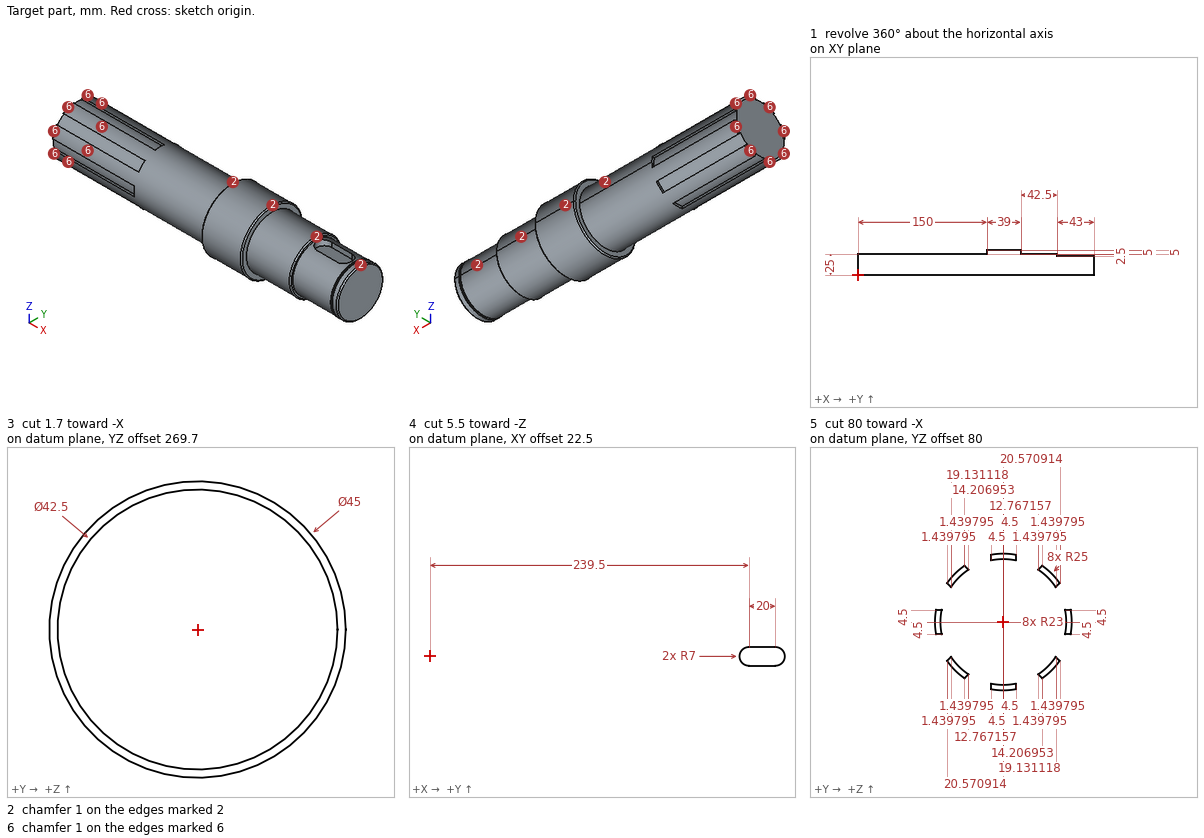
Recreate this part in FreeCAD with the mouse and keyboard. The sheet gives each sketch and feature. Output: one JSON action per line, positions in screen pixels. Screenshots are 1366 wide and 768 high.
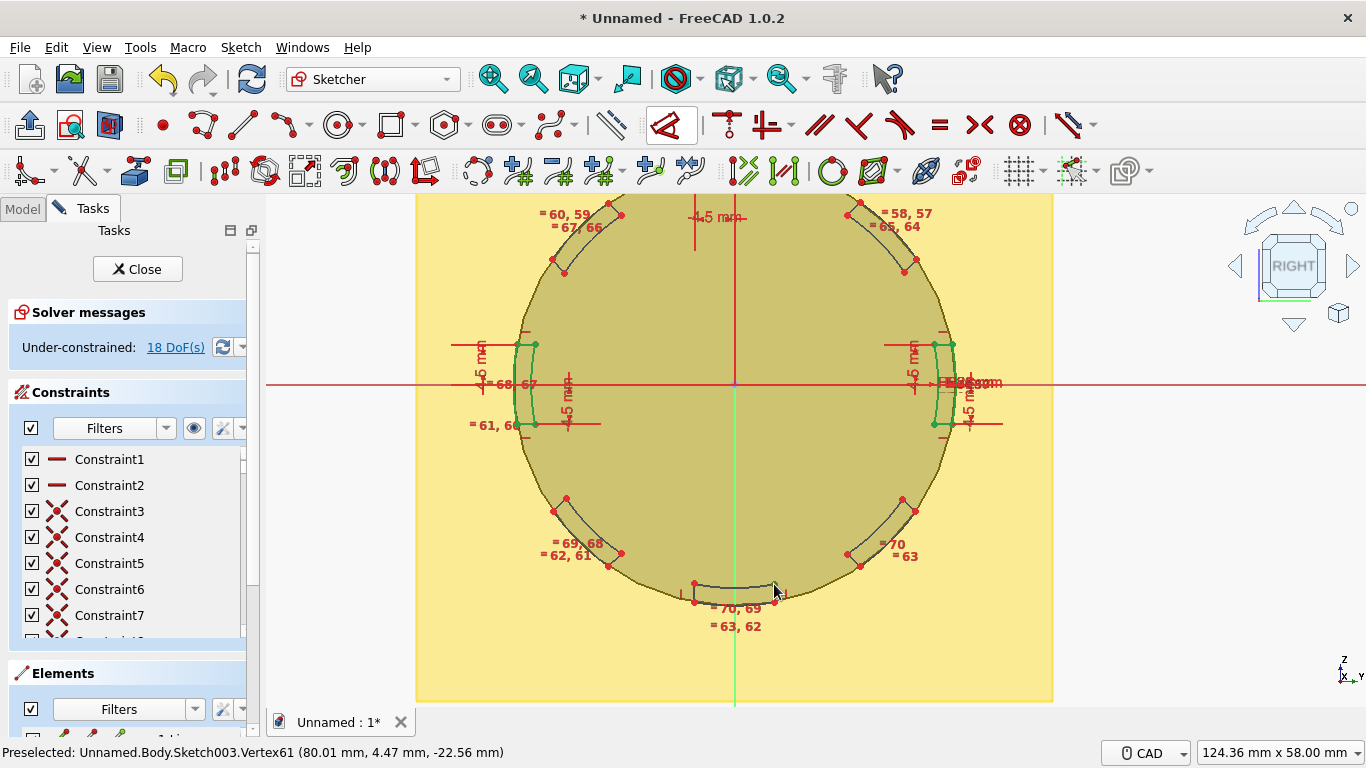
{"action": "key", "text": "l"}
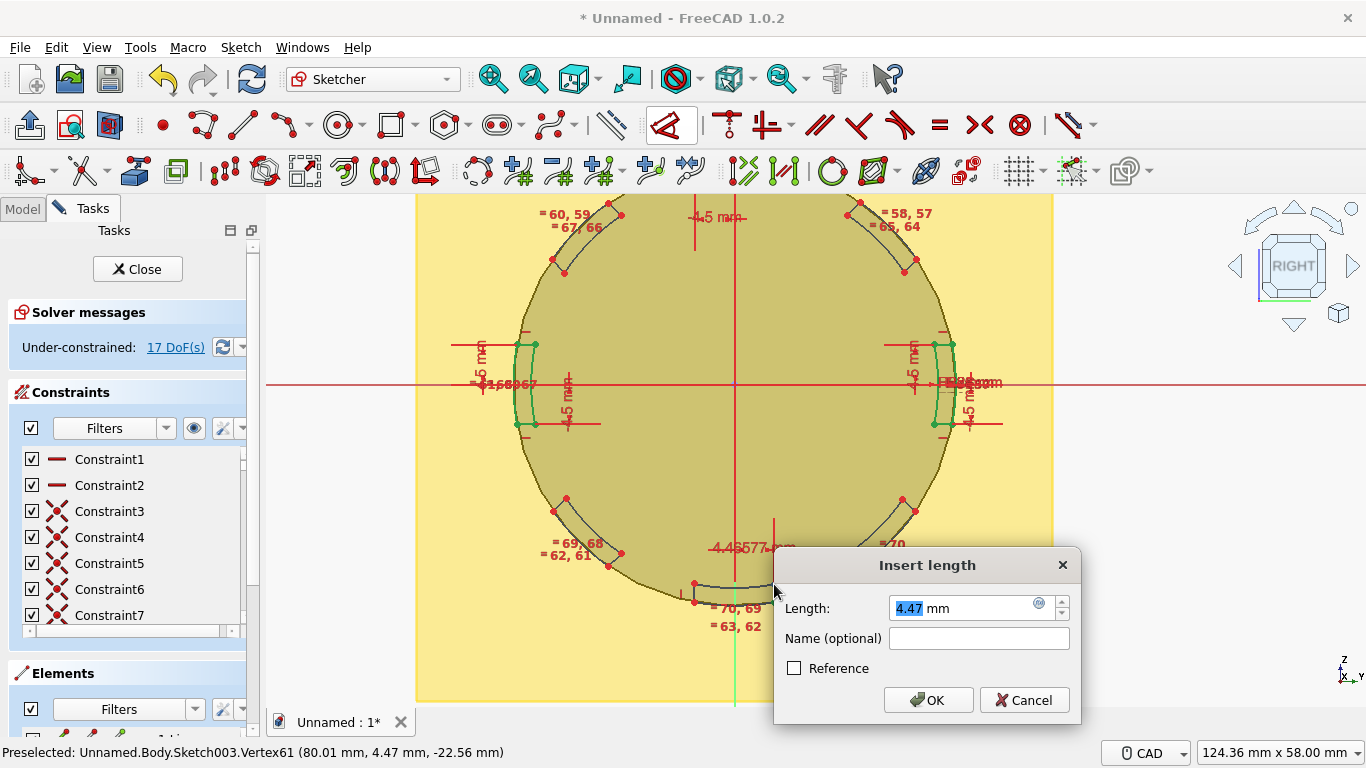
{"action": "type", "text": "4.5"}
{"action": "key", "text": "Return"}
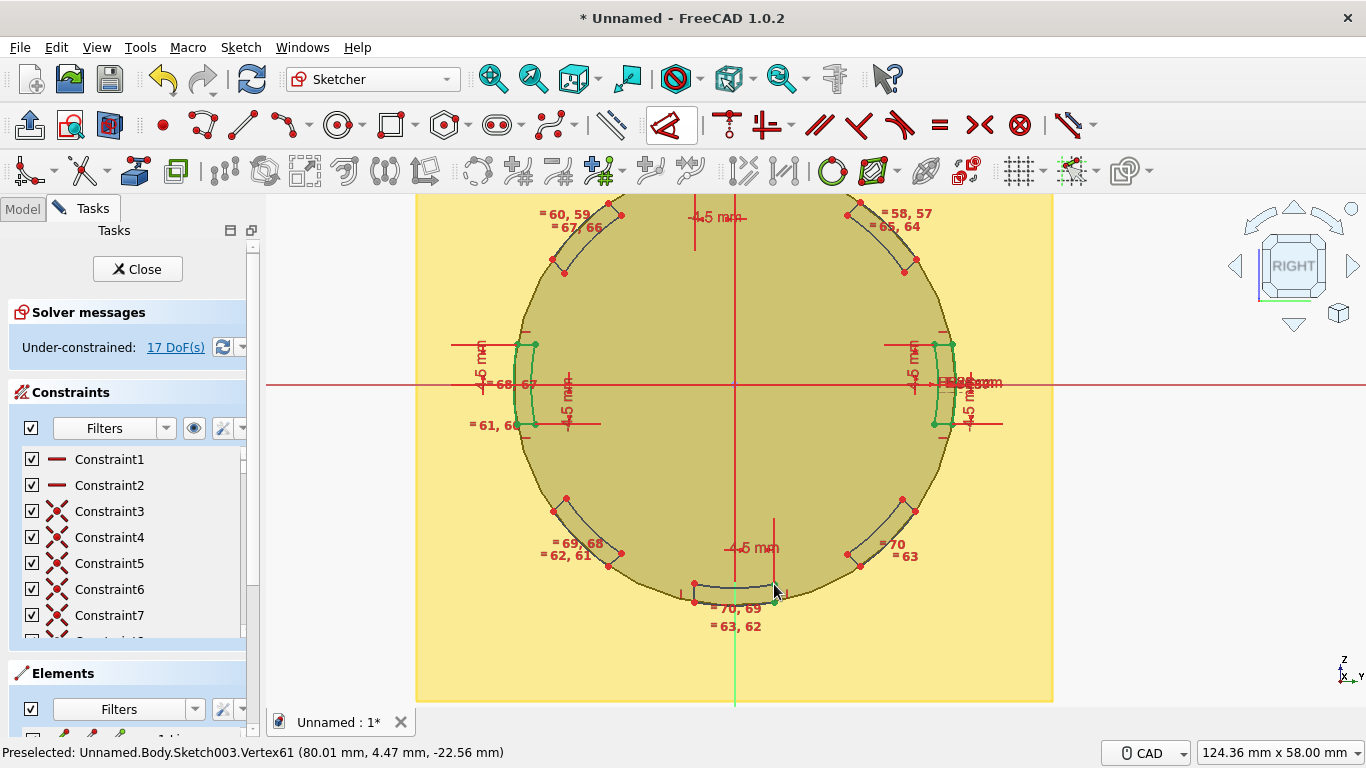
{"action": "left_click", "coordinate": [694, 602]}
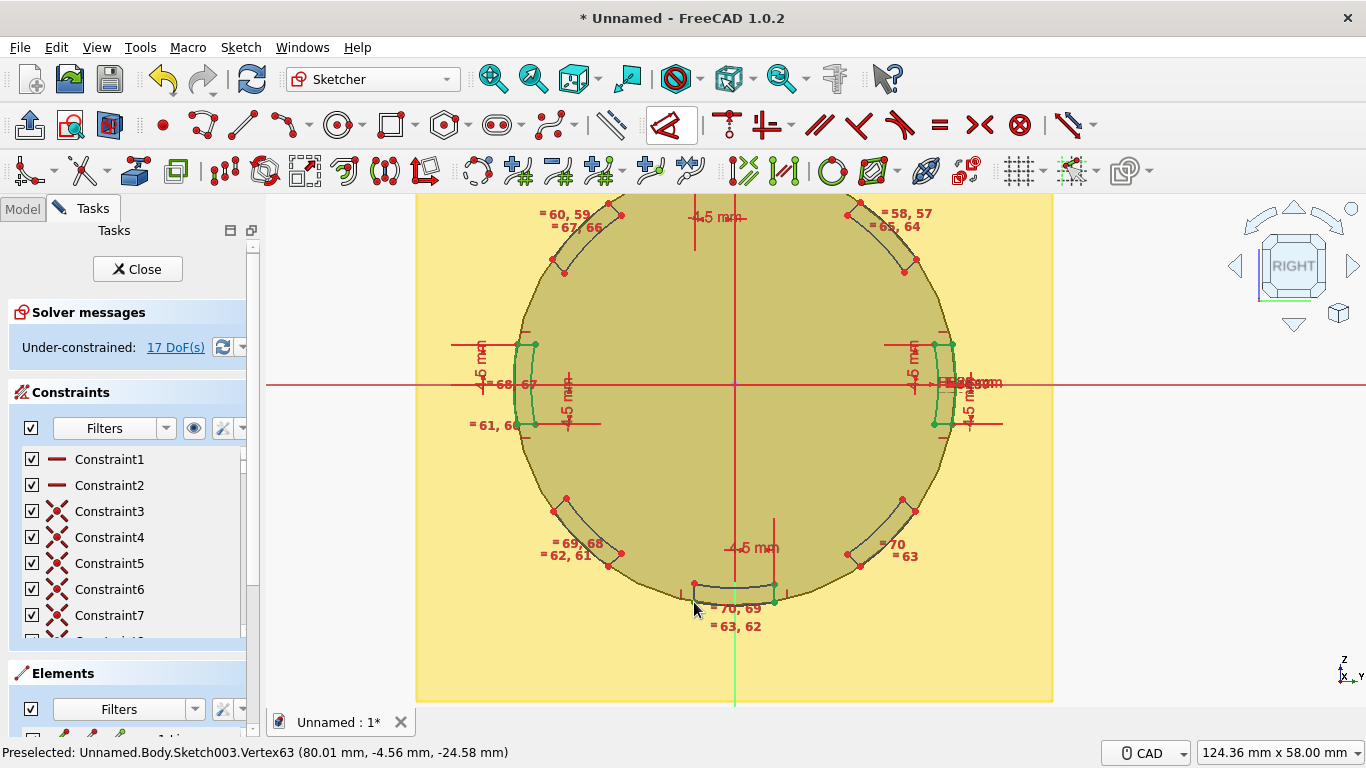
{"action": "key", "text": "l"}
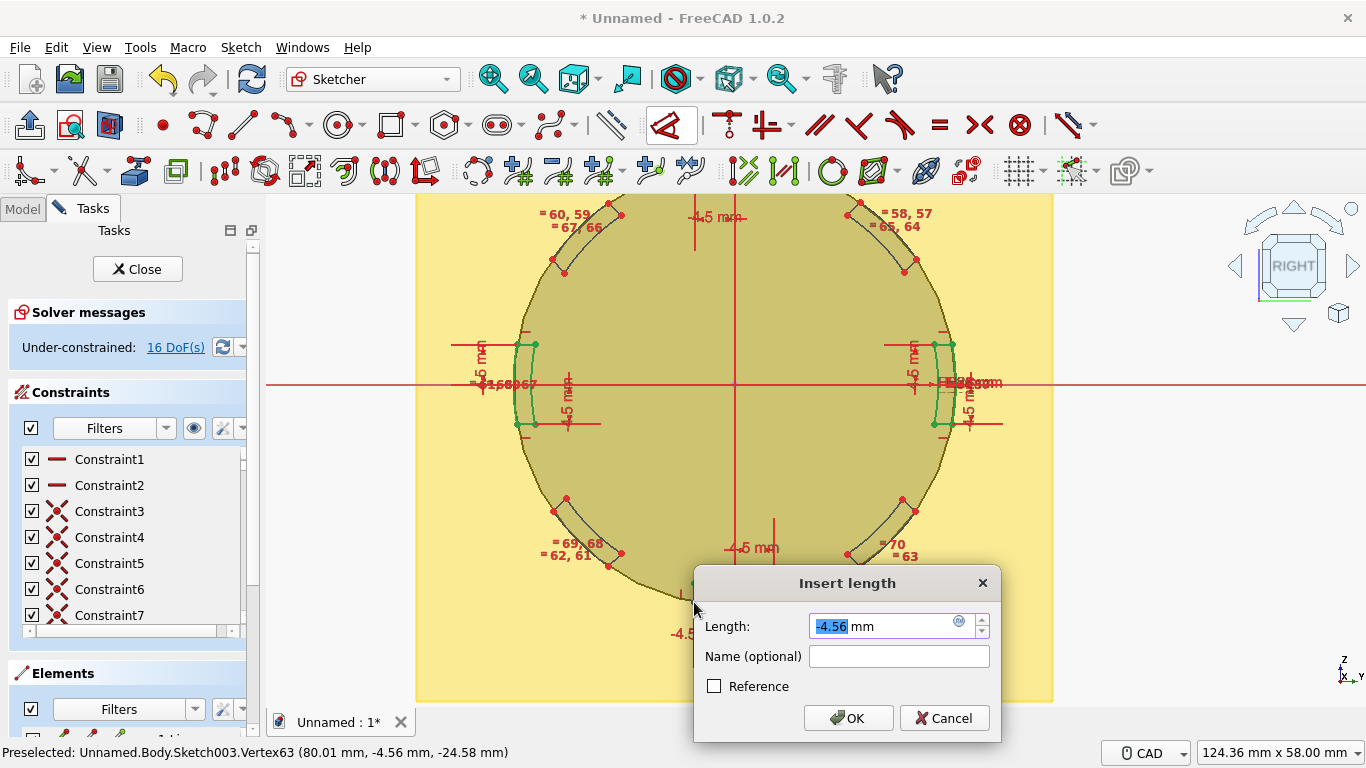
{"action": "type", "text": "-4.5"}
{"action": "key", "text": "Return"}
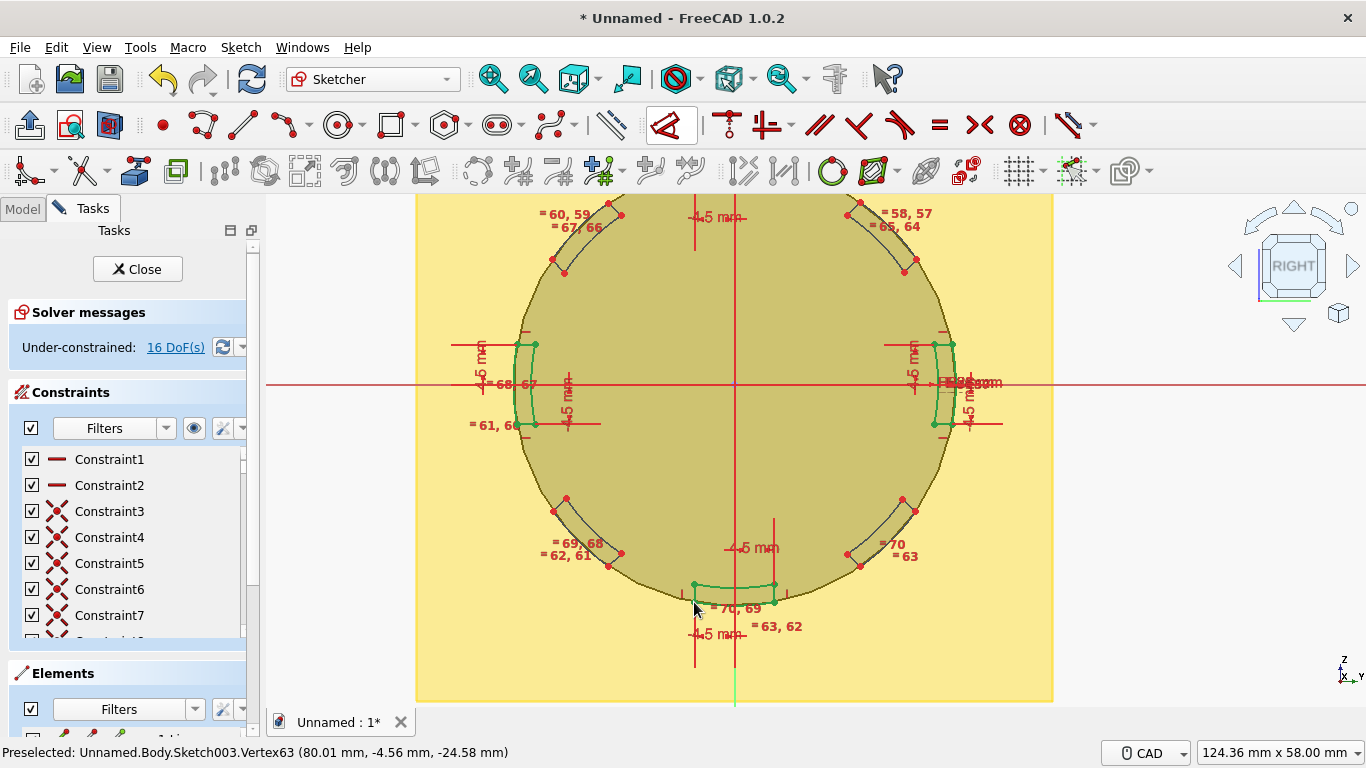
{"action": "scroll", "coordinate": [774, 585], "scroll_direction": "down", "scroll_amount": 2}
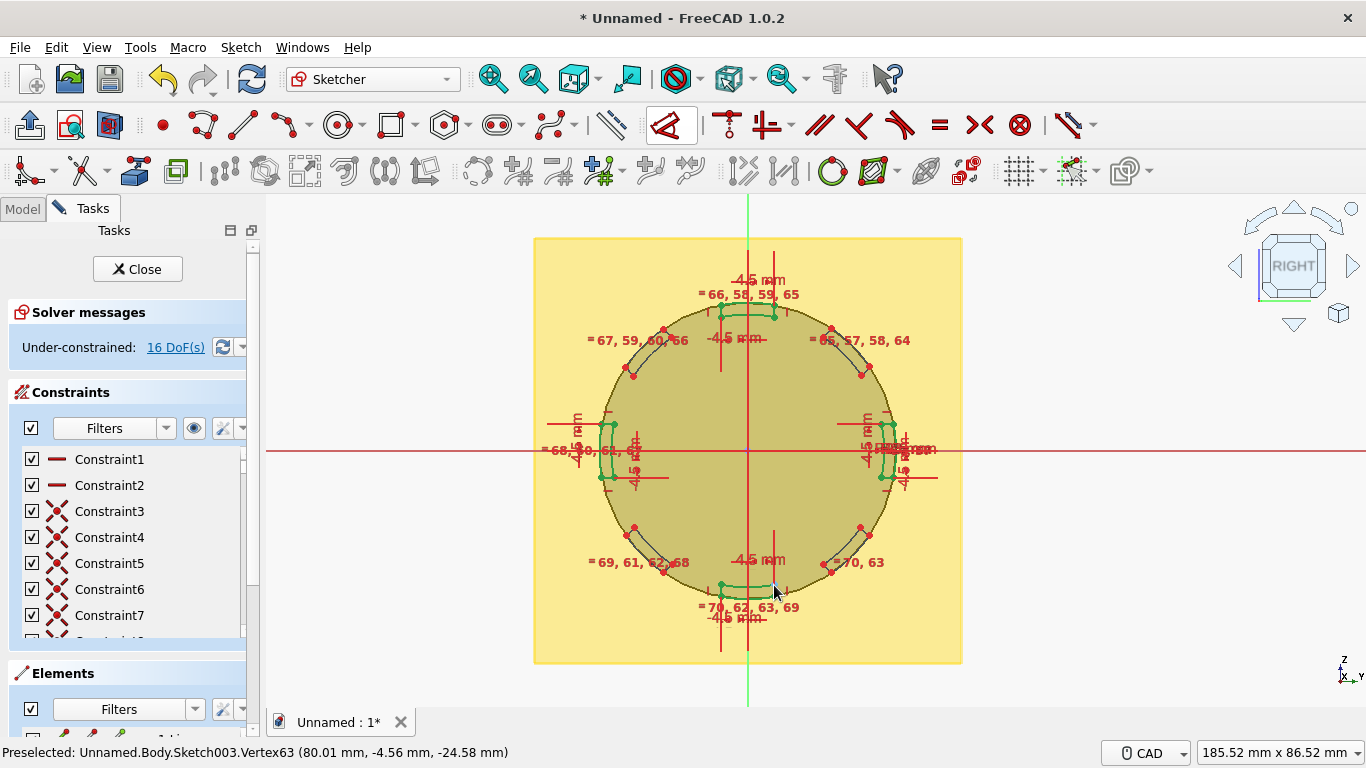
{"action": "scroll", "coordinate": [828, 333], "scroll_direction": "up", "scroll_amount": 8}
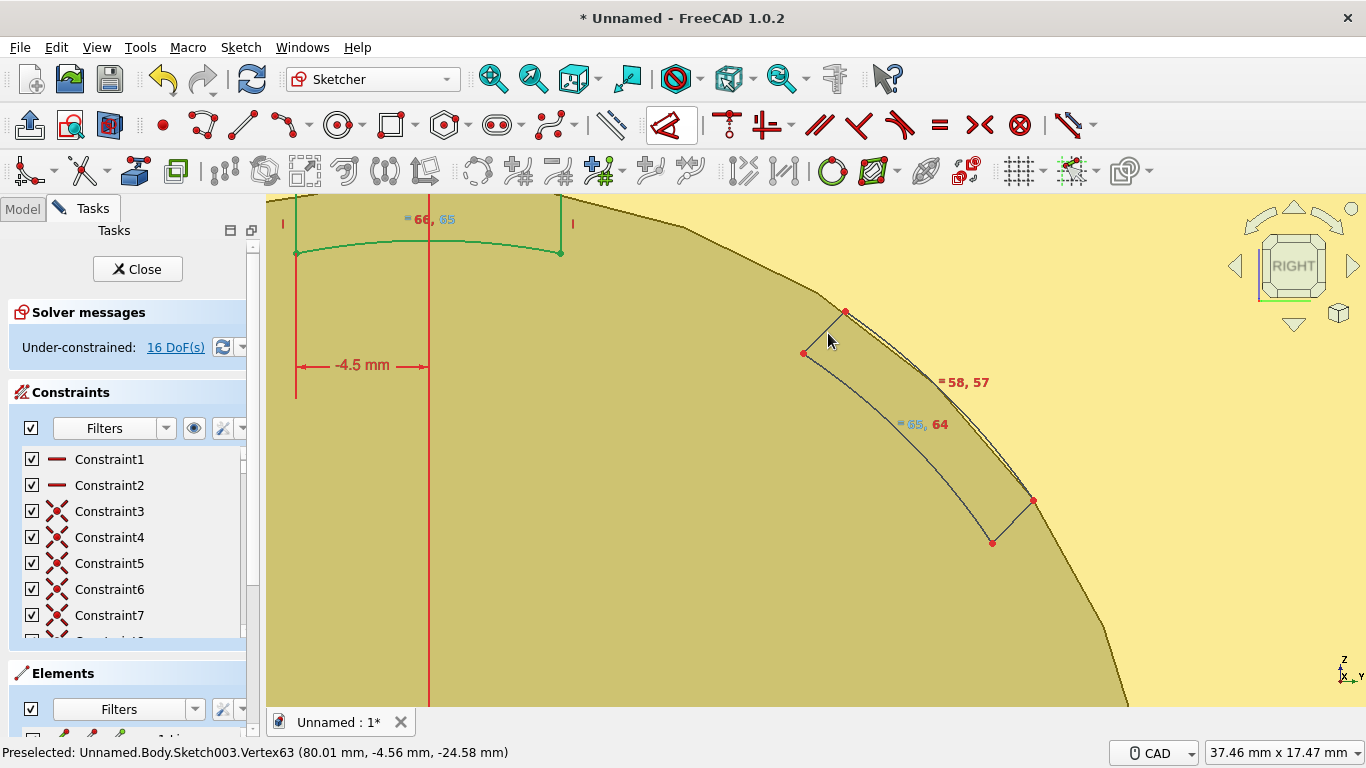
{"action": "left_click", "coordinate": [824, 333]}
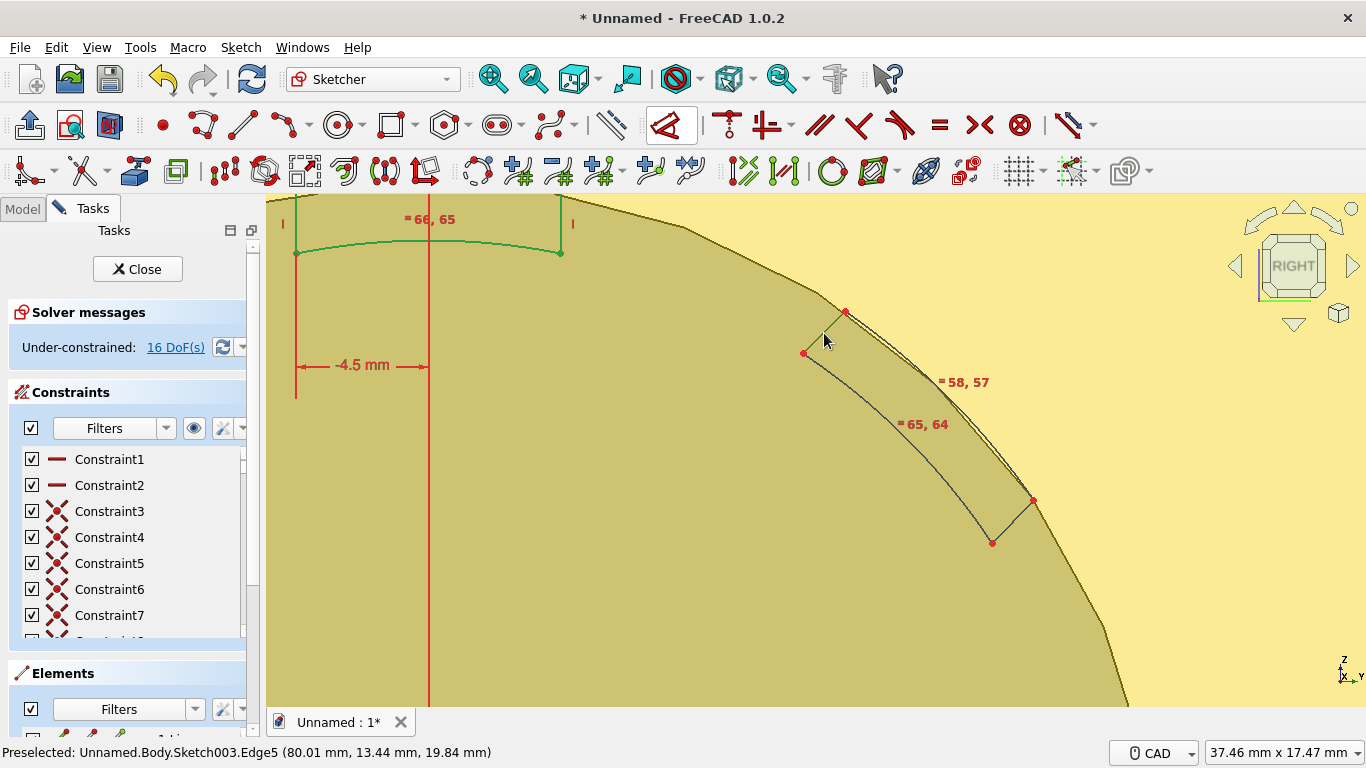
{"action": "left_click", "coordinate": [692, 126]}